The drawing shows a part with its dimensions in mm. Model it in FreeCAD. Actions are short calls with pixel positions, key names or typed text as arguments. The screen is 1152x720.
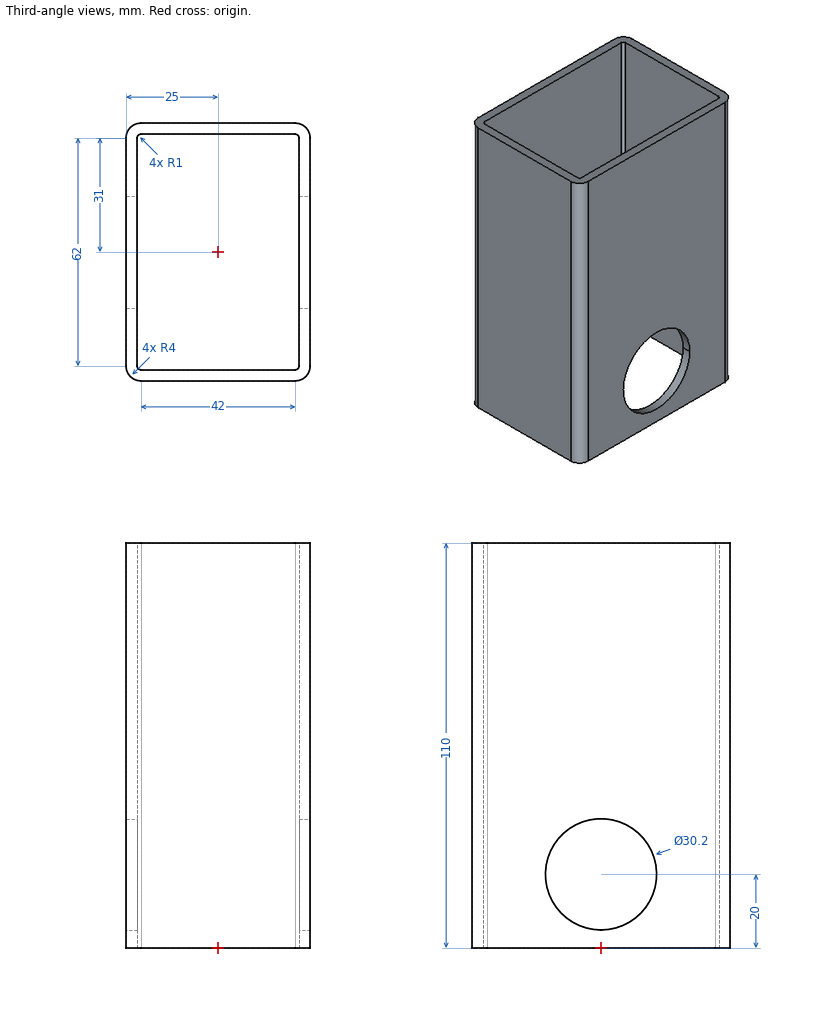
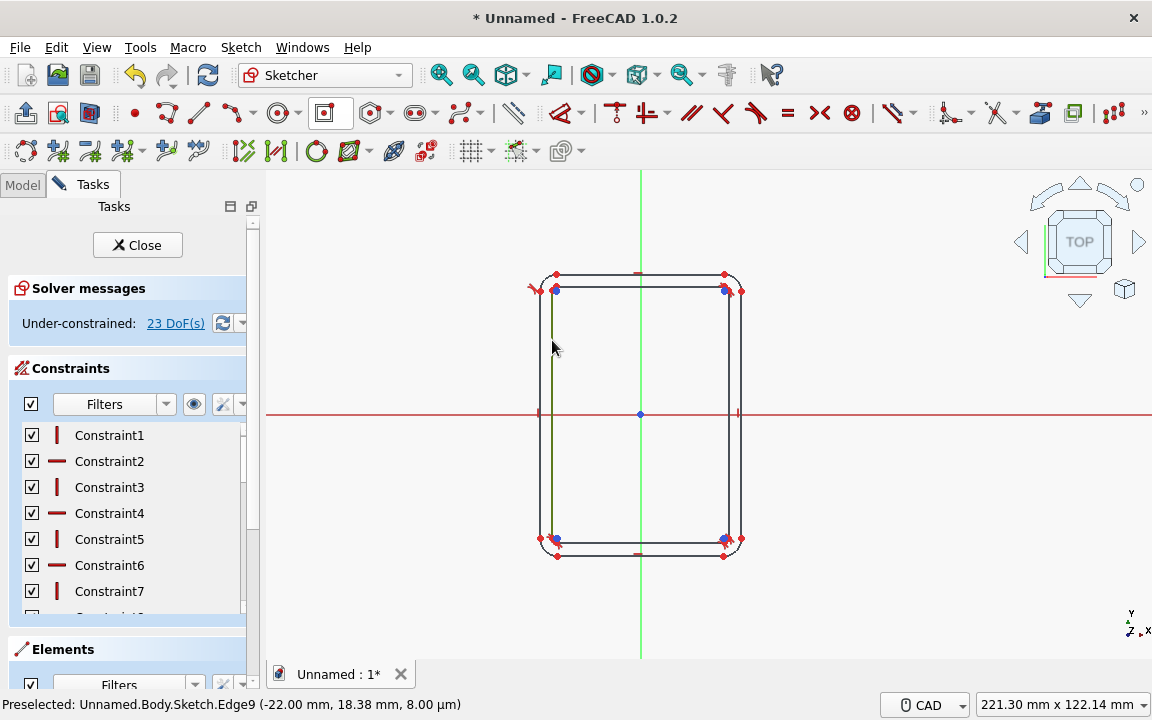
scroll(554, 542, up, 8)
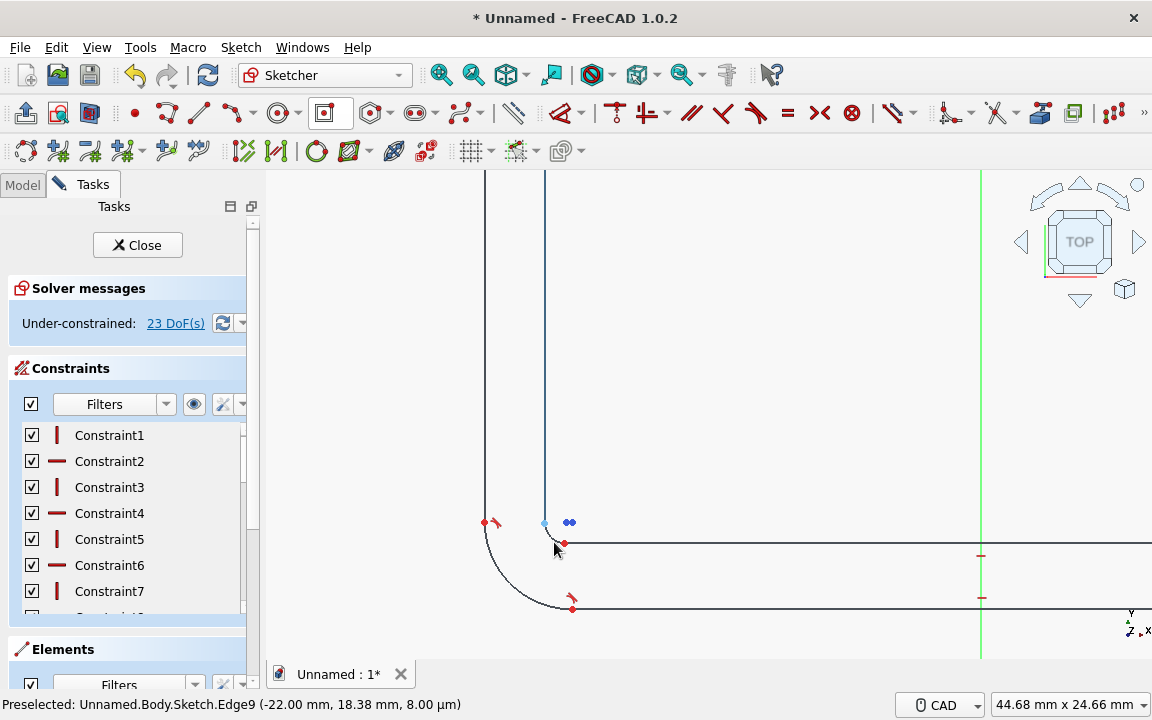
click(551, 537)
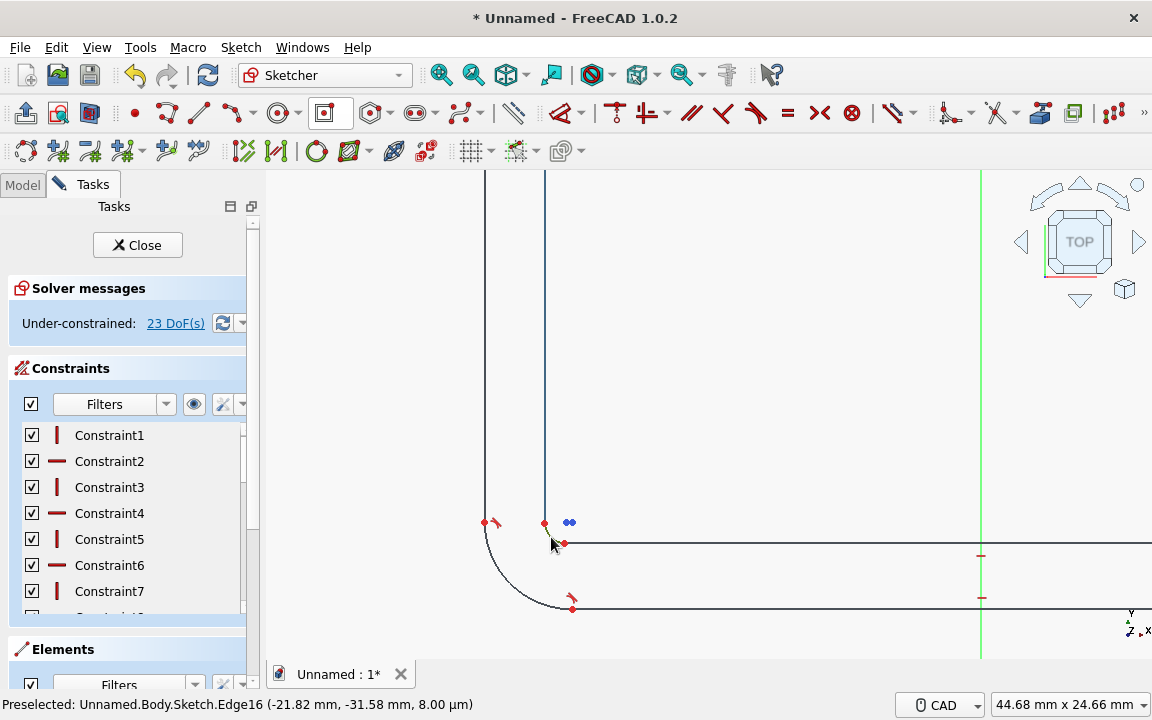
click(756, 114)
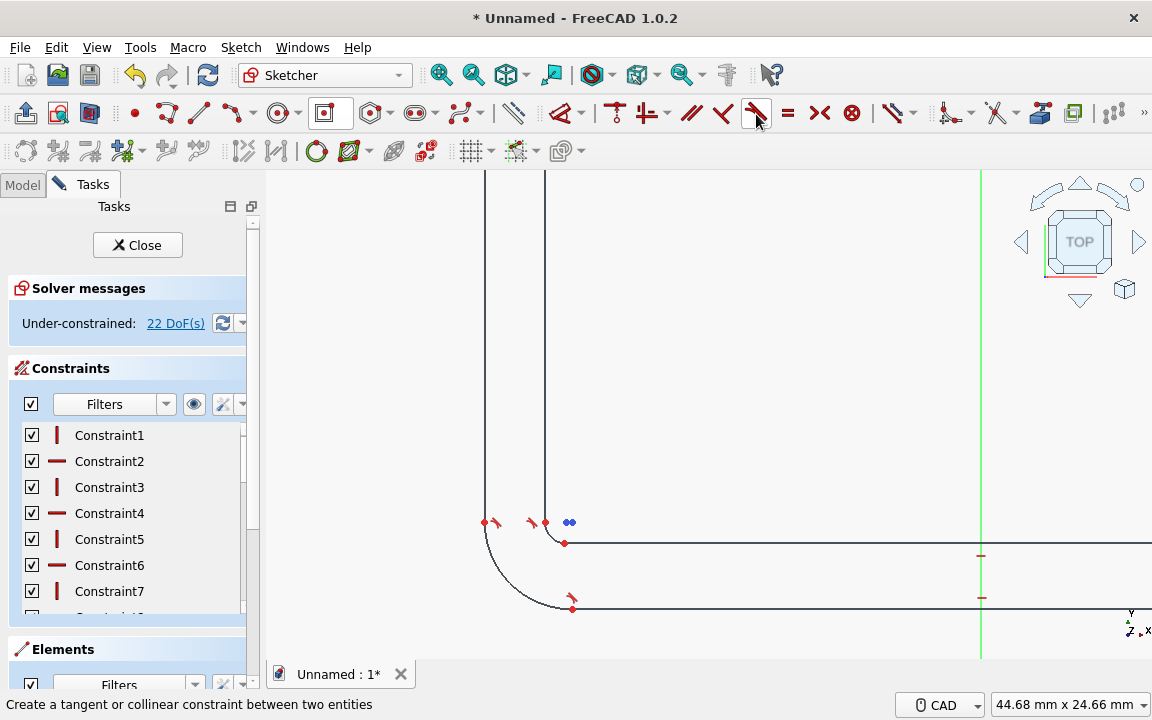
scroll(554, 543, down, 8)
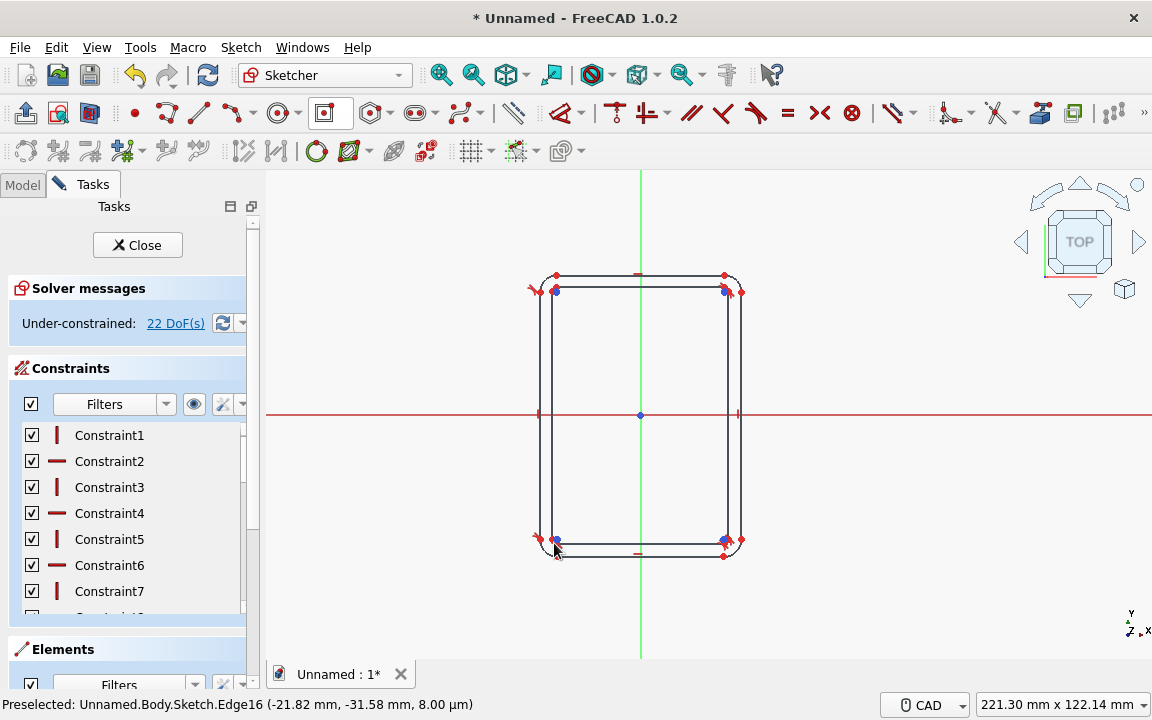
click(607, 287)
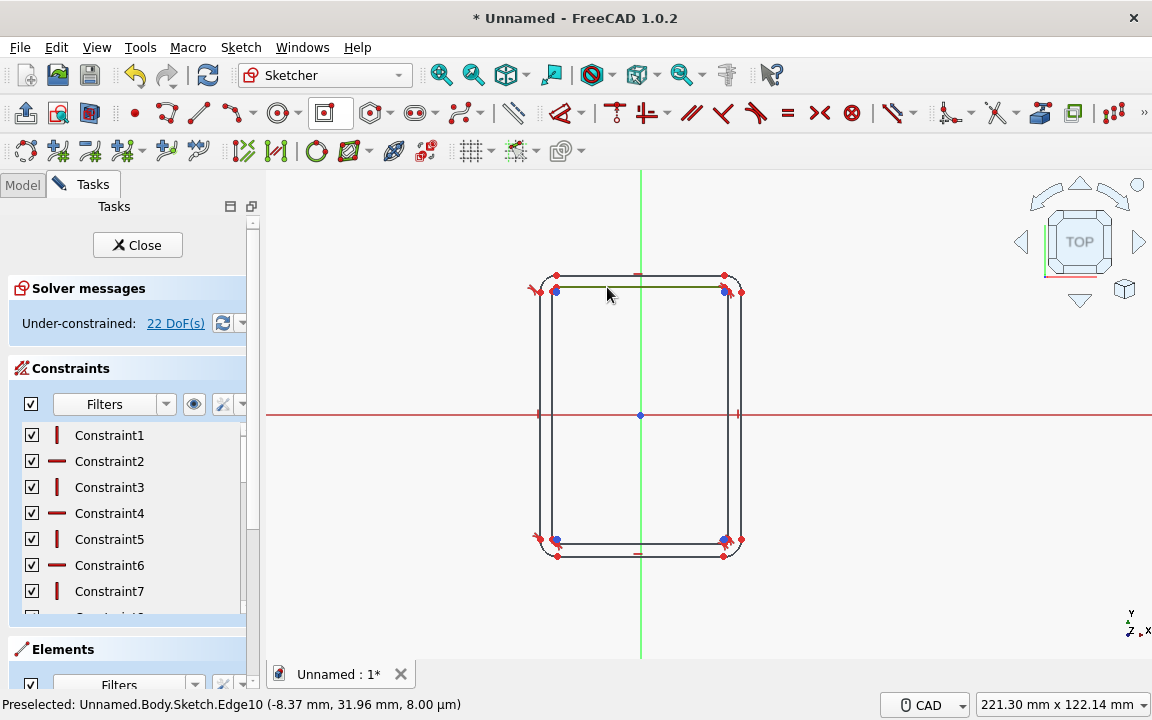
scroll(554, 289, up, 8)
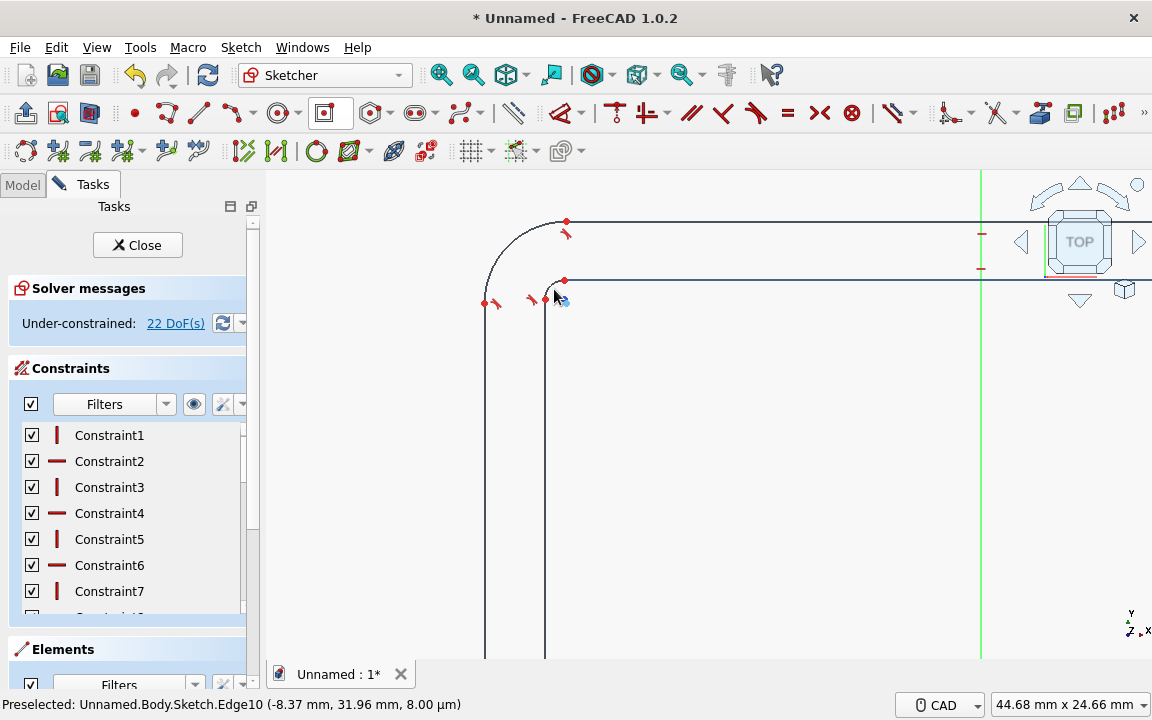
click(551, 286)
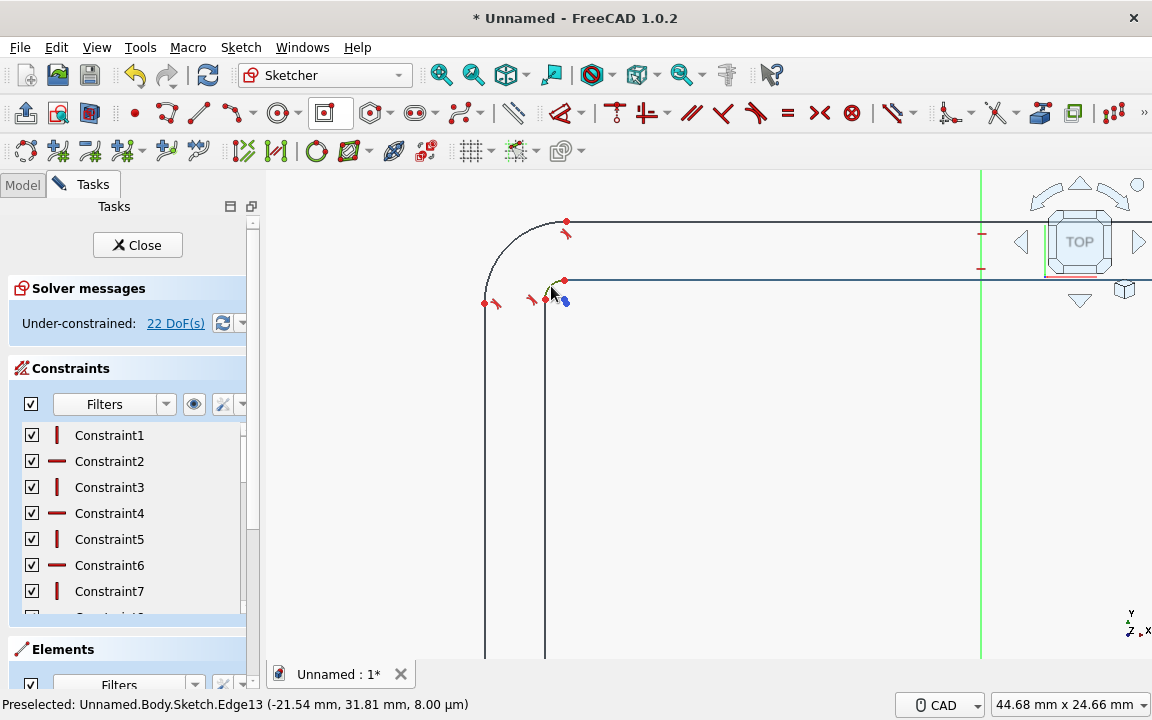
key(t)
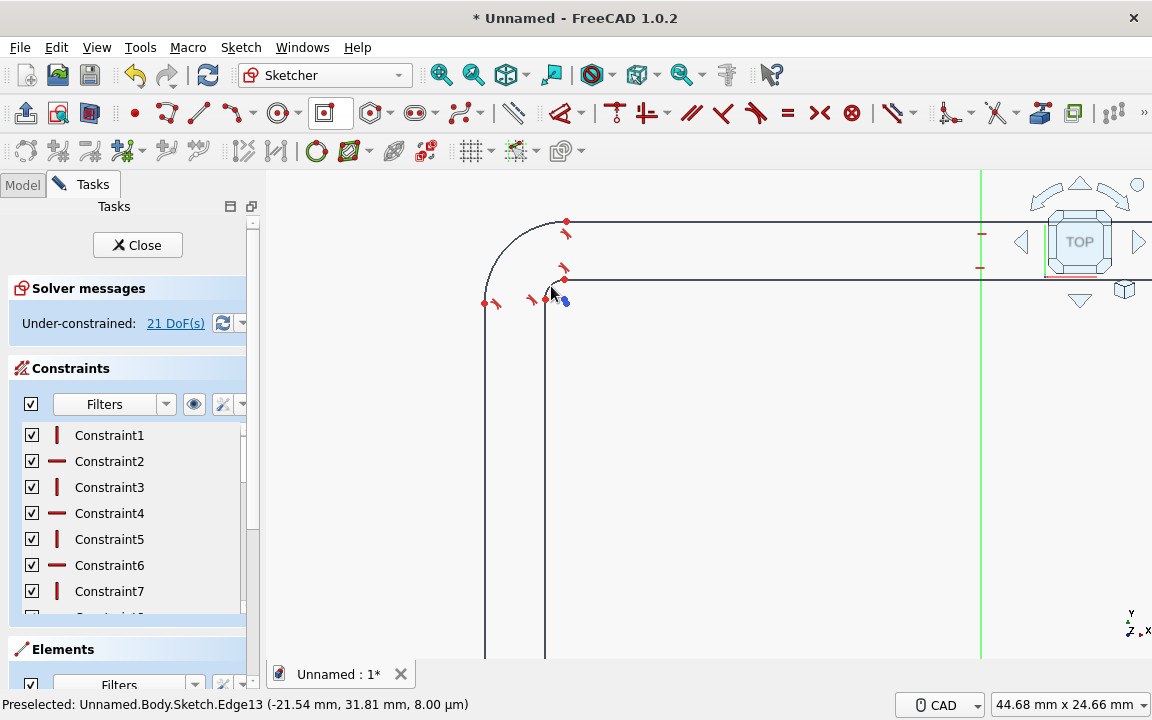
scroll(554, 288, down, 8)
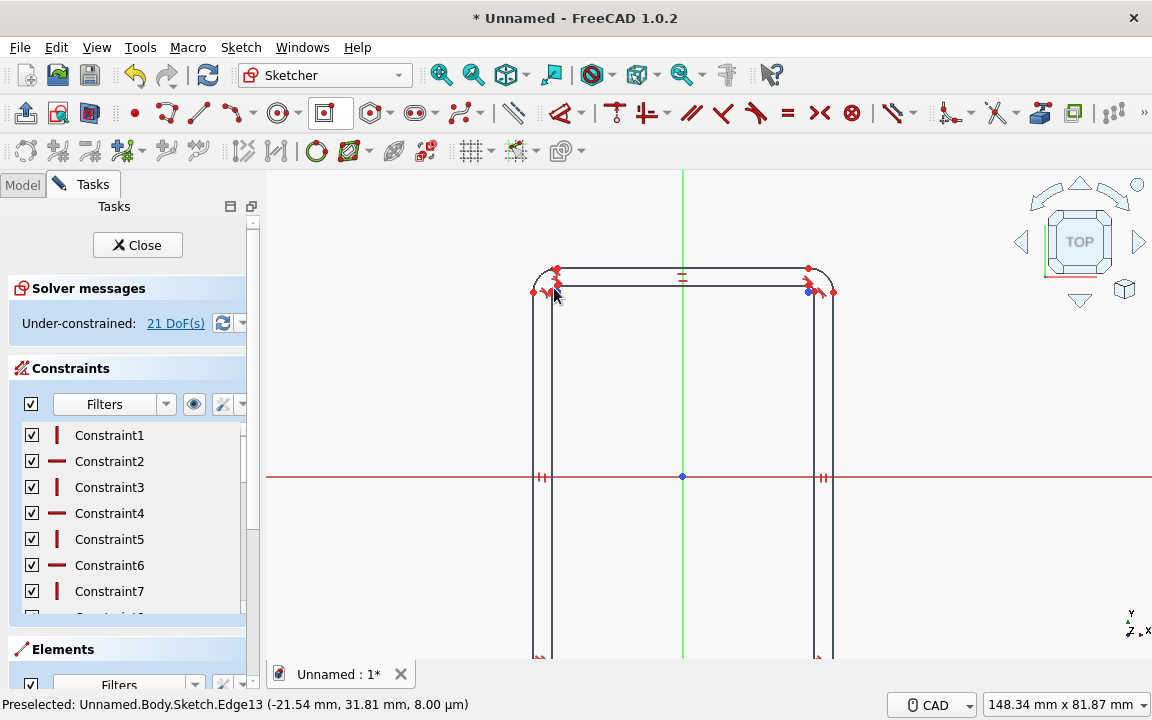
click(607, 287)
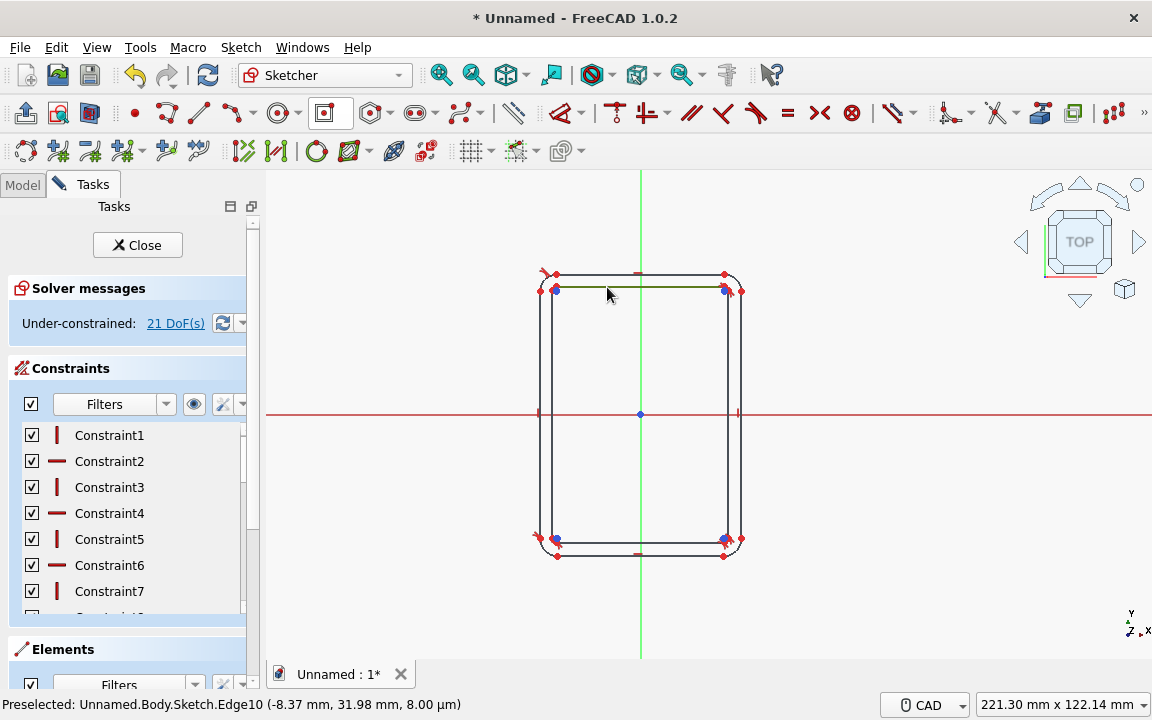
scroll(727, 288, up, 8)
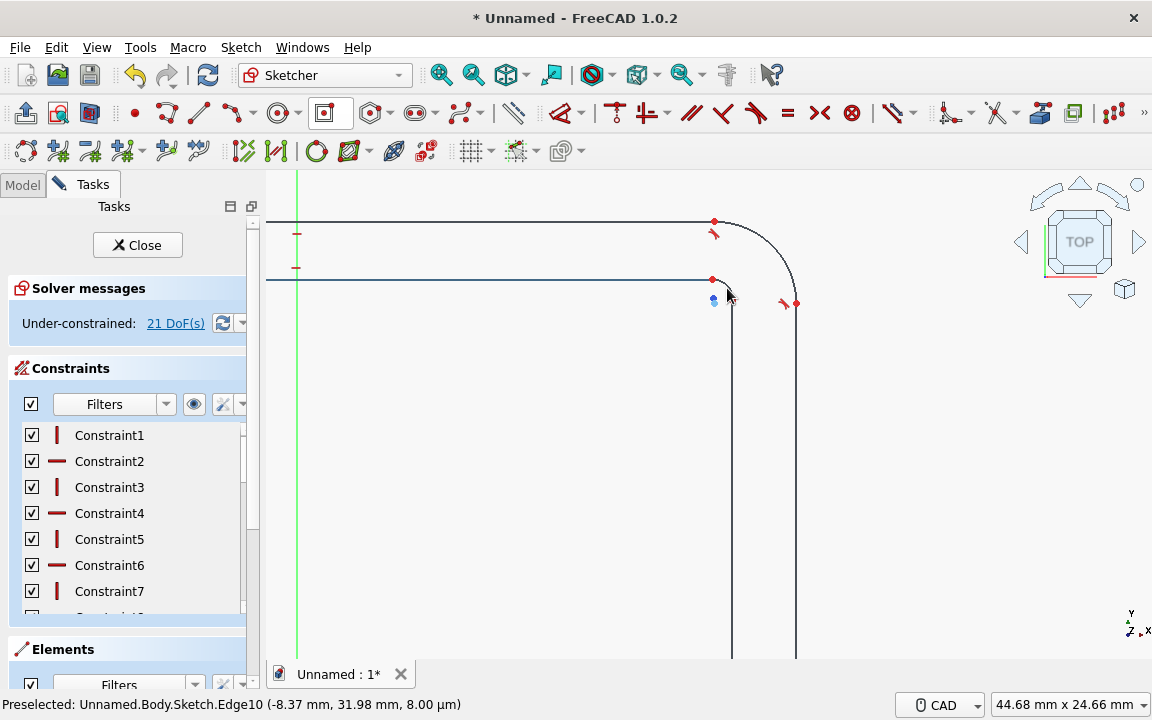
click(727, 286)